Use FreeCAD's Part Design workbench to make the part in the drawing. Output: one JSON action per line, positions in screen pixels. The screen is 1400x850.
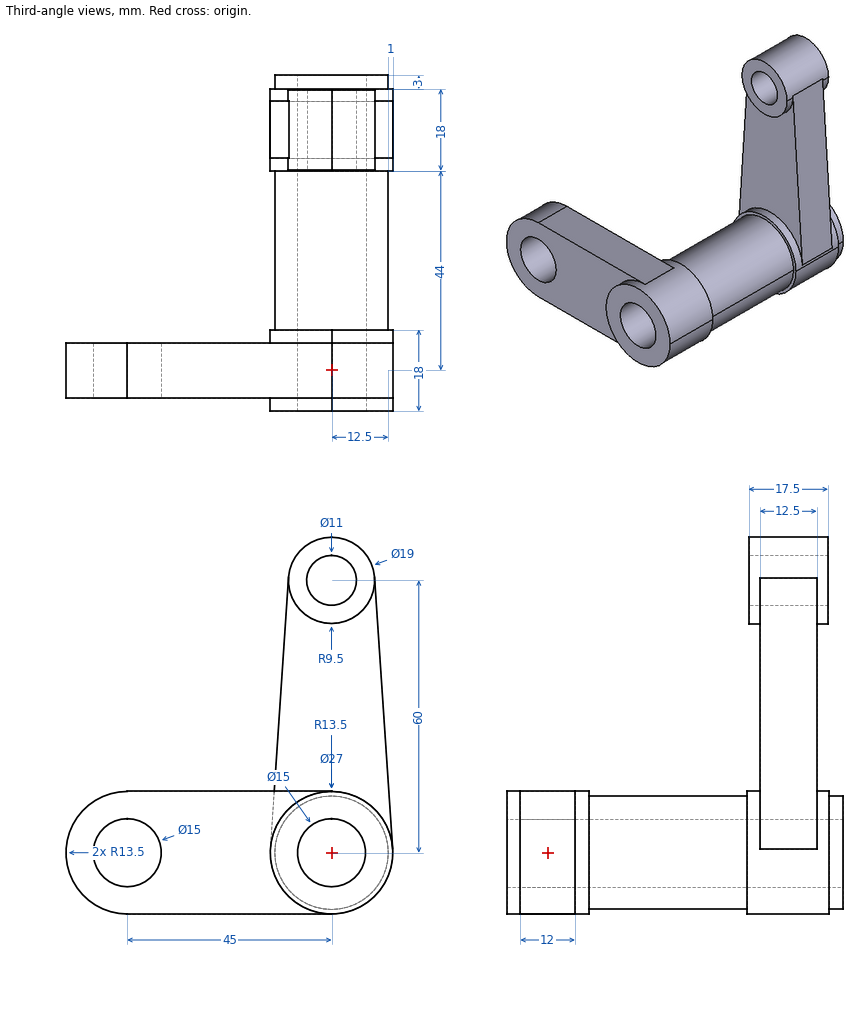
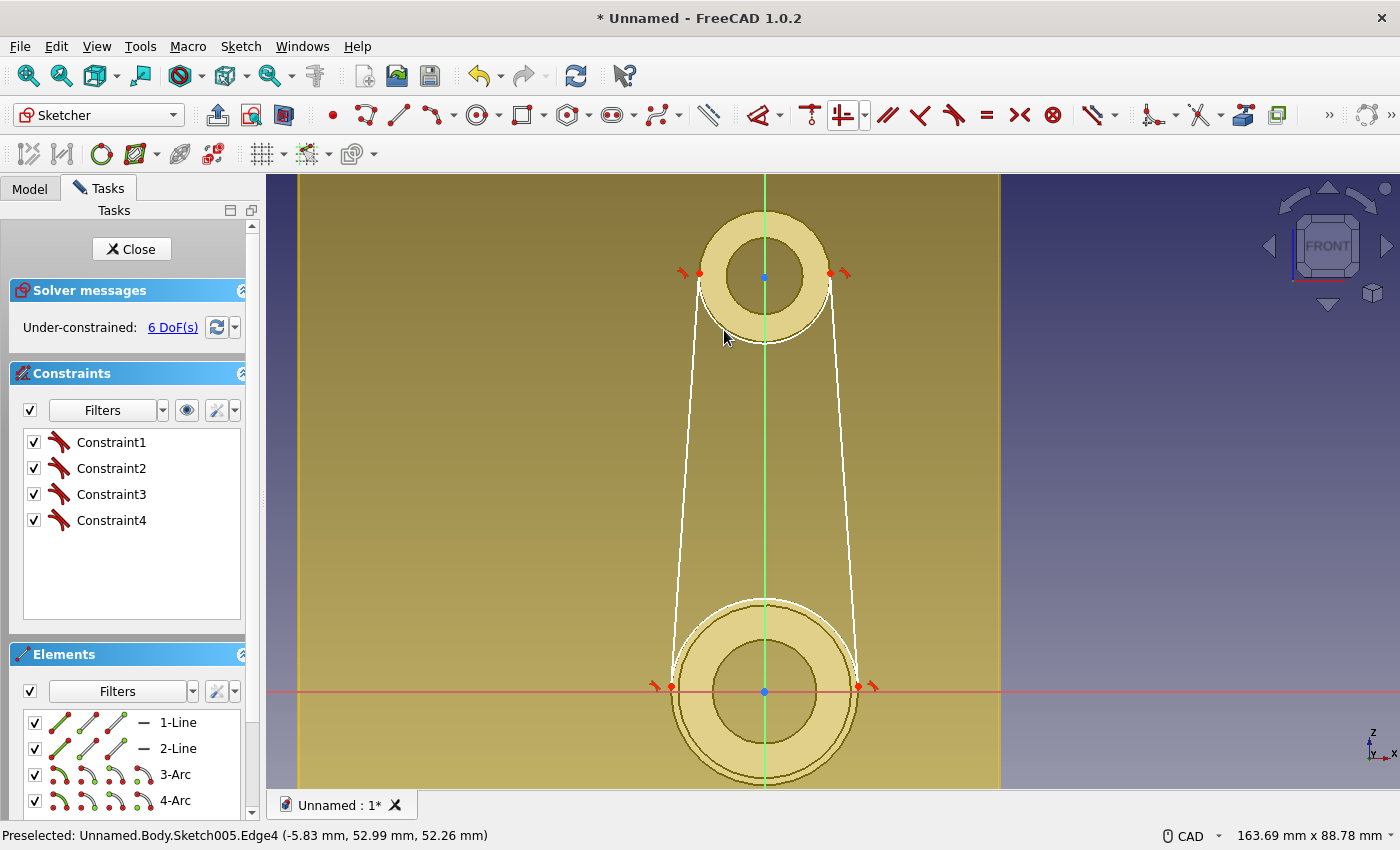
{"action": "left_click_drag", "start_coordinate": [755, 682], "coordinate": [775, 702]}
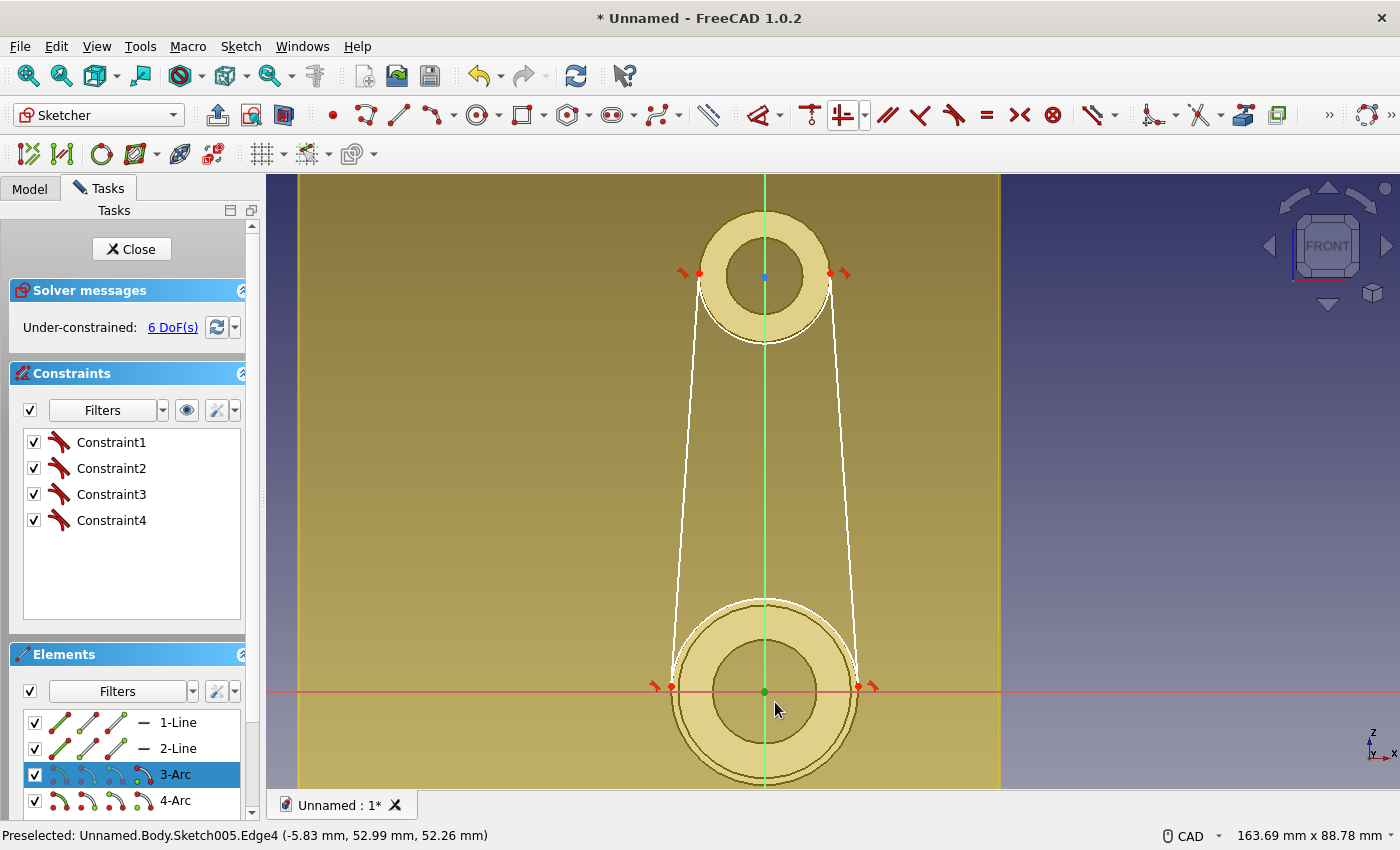
{"action": "left_click", "coordinate": [810, 116]}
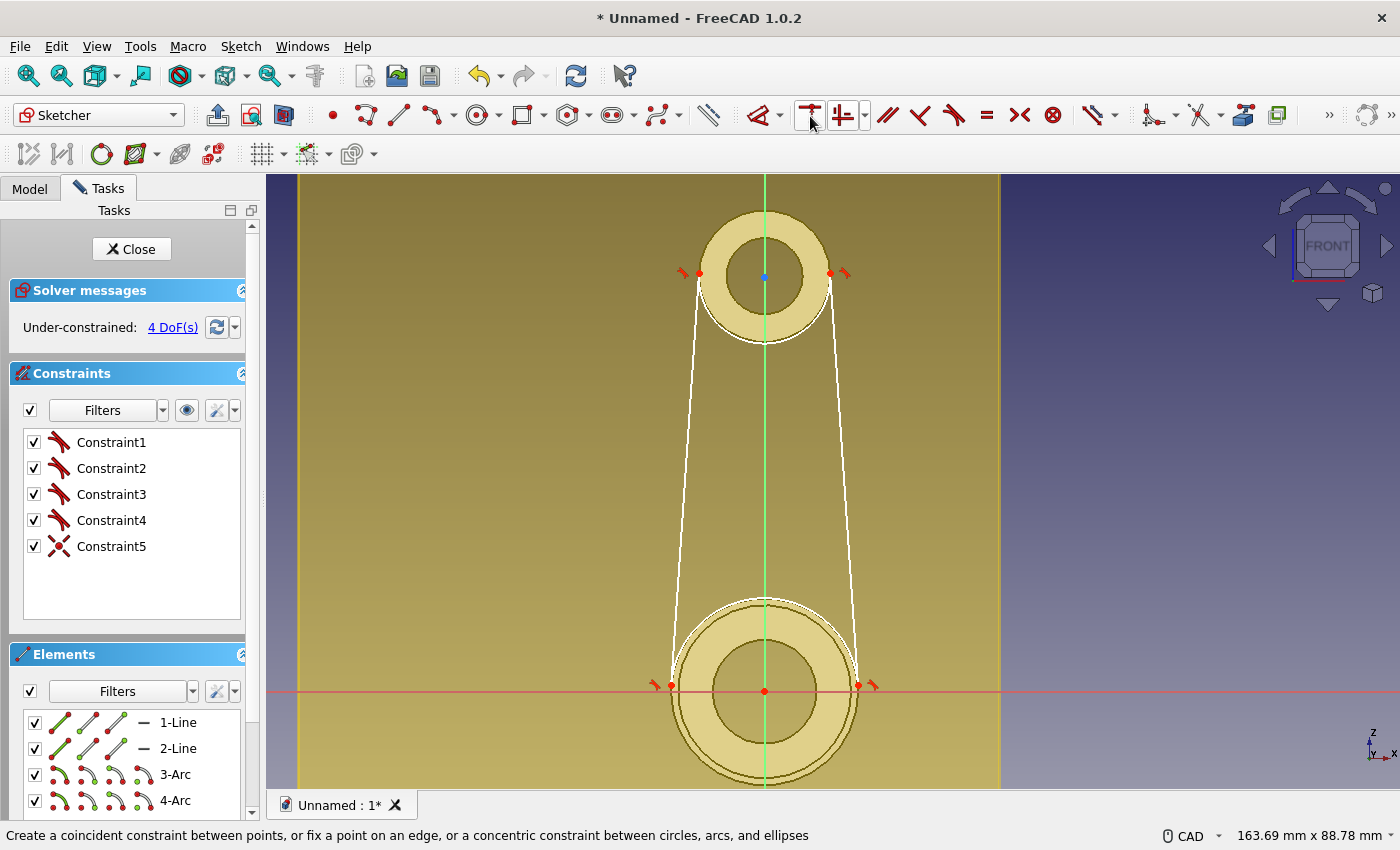
{"action": "left_click", "coordinate": [765, 278]}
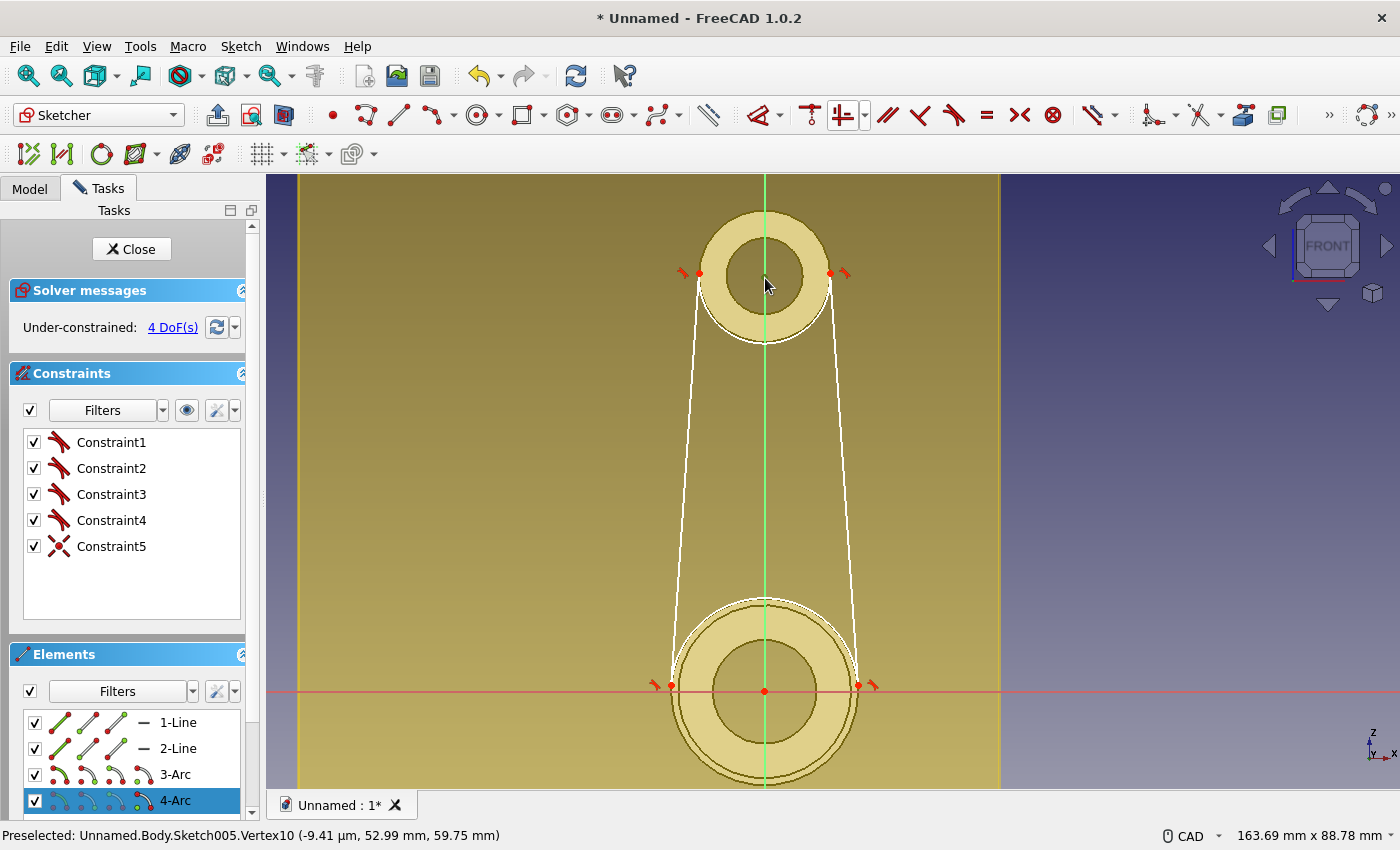
{"action": "left_click", "coordinate": [765, 641]}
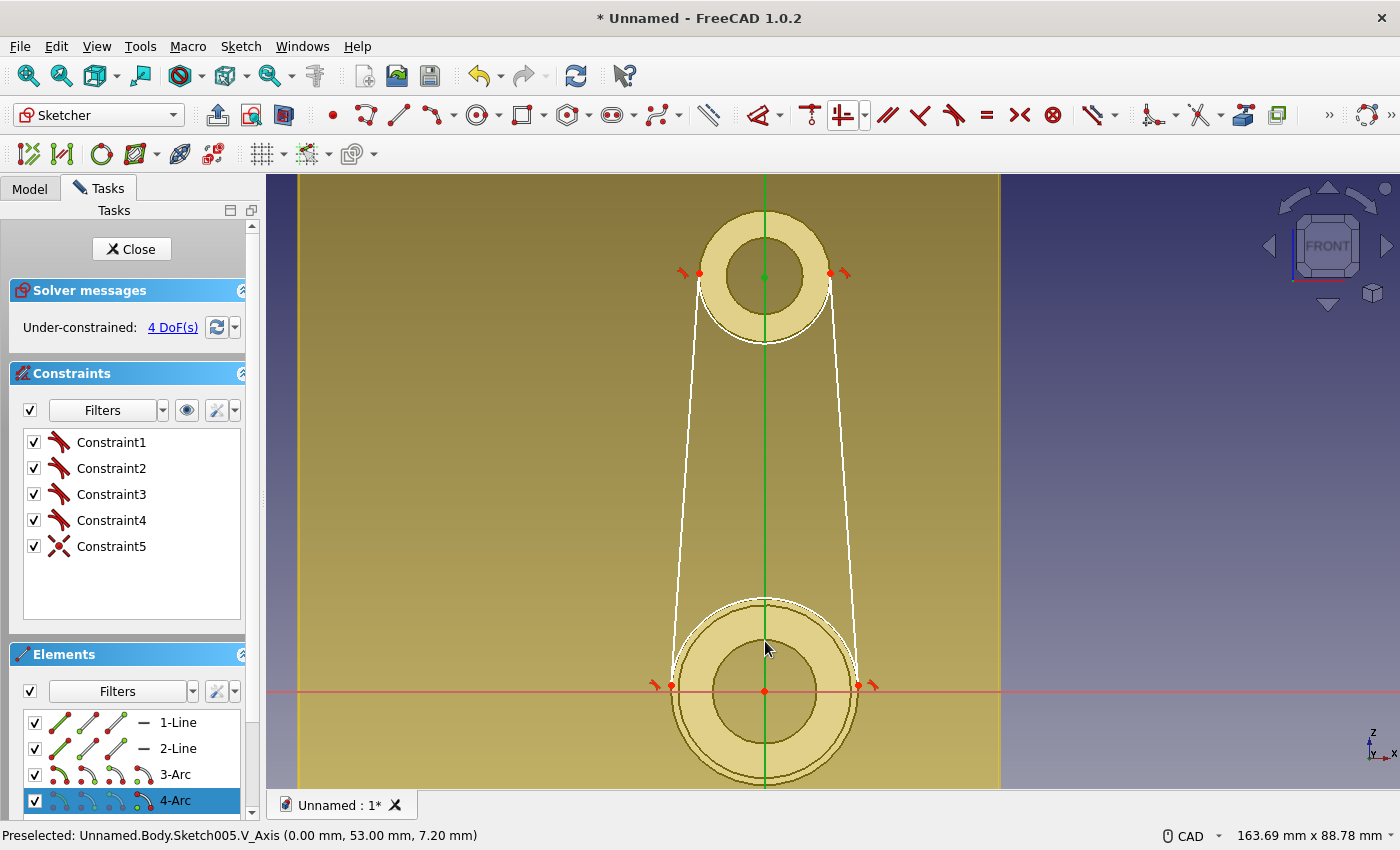
{"action": "key", "text": "c"}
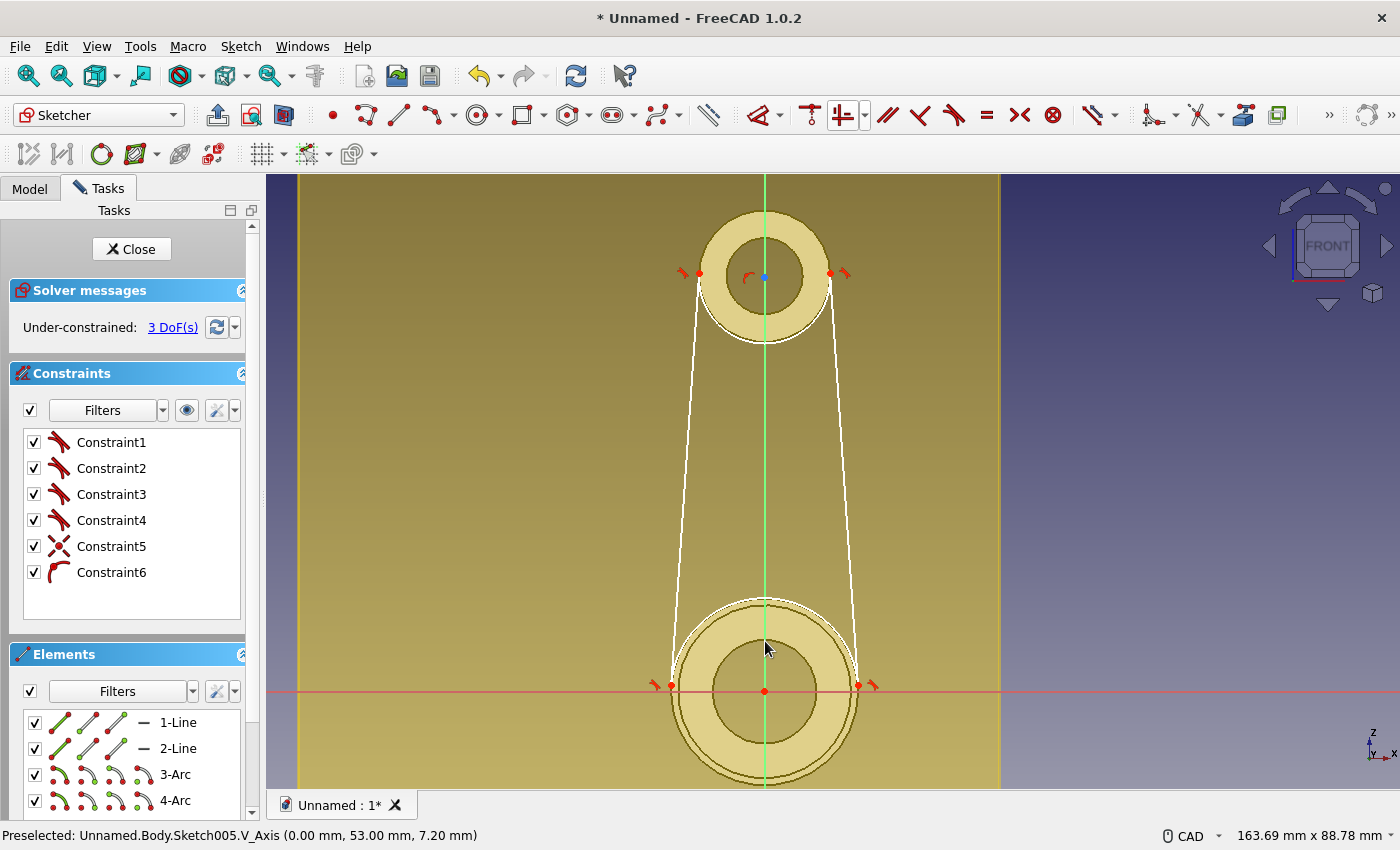
{"action": "key", "text": "d"}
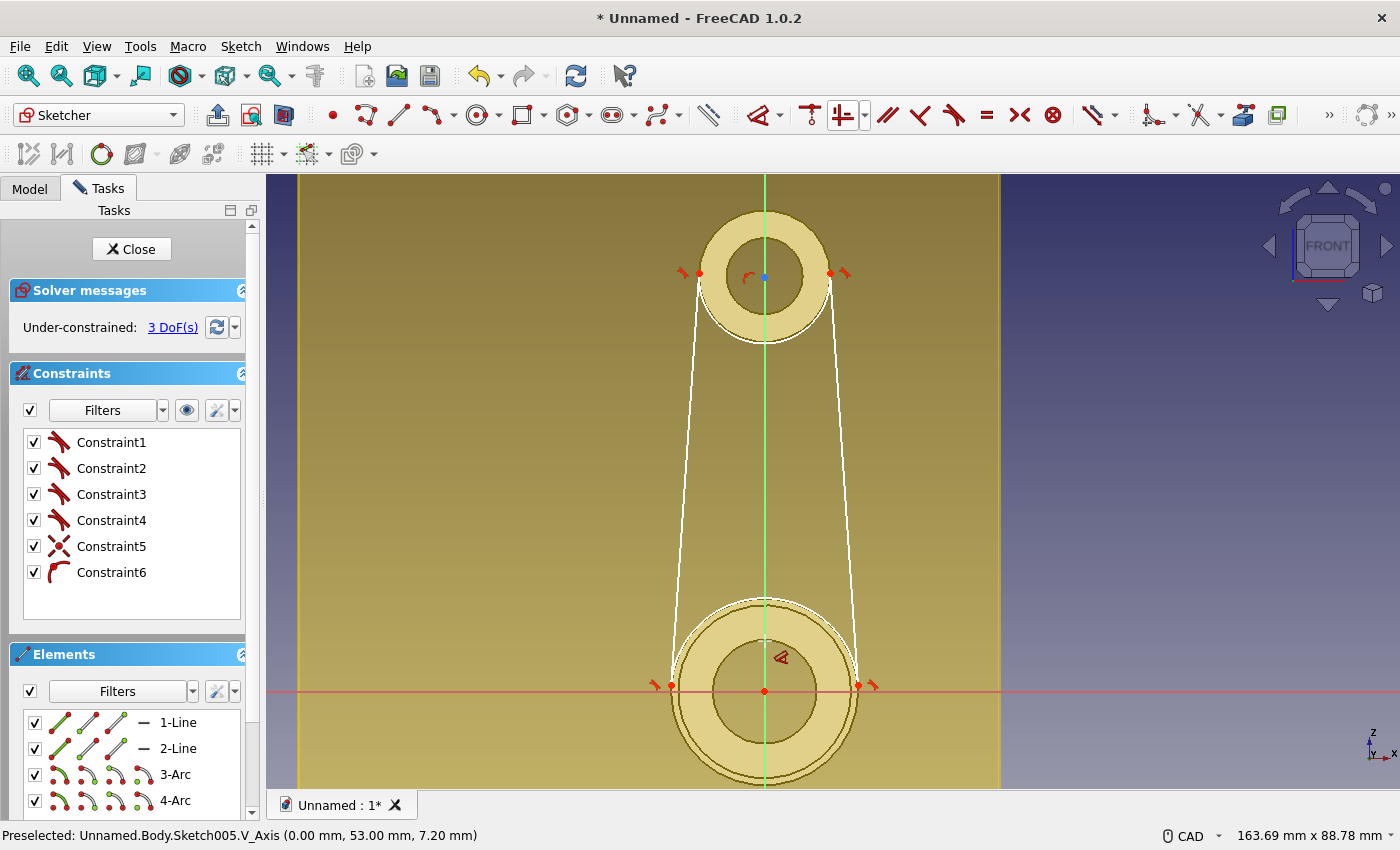
{"action": "left_click", "coordinate": [818, 615]}
{"action": "left_click", "coordinate": [836, 589]}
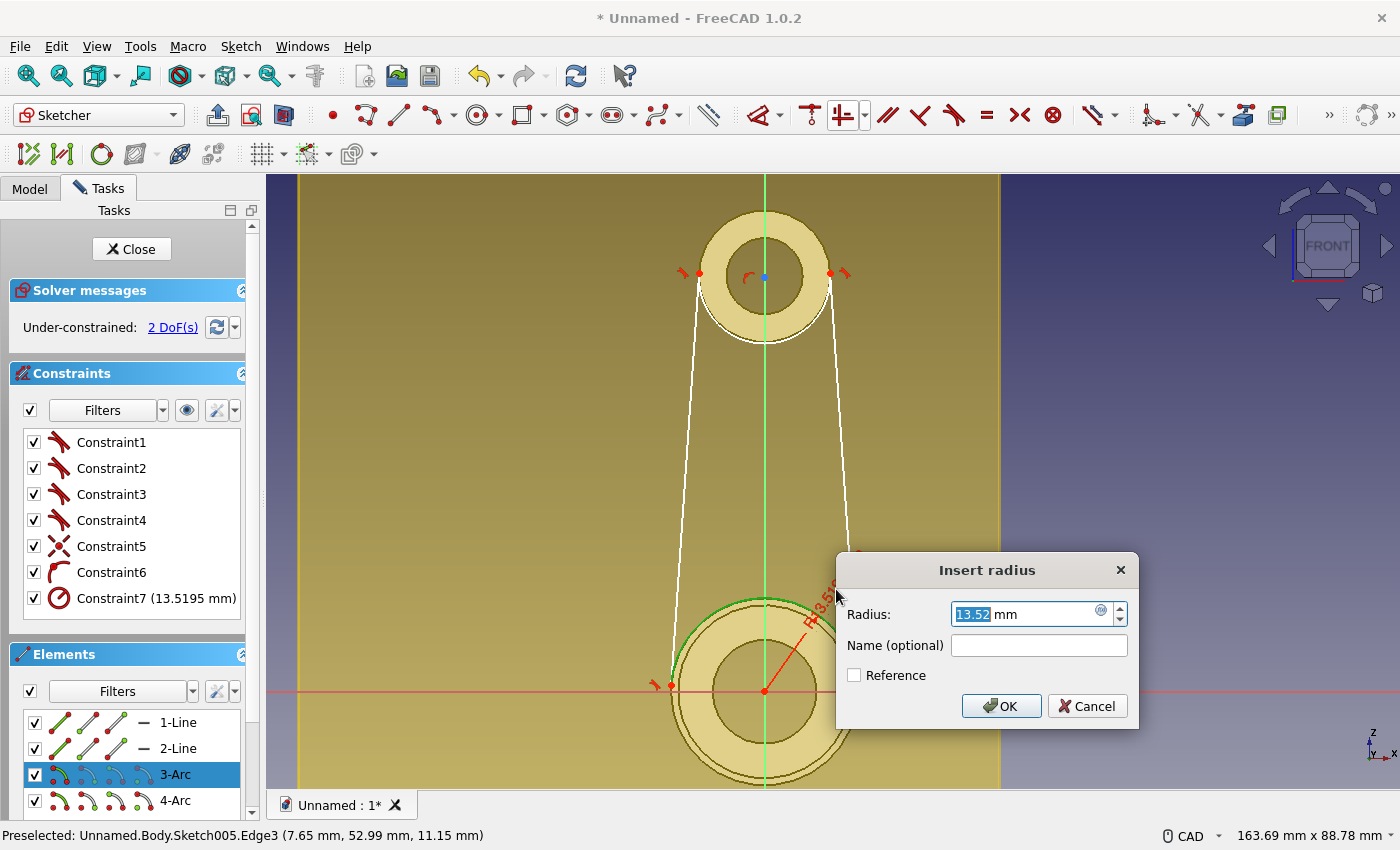
{"action": "type", "text": "13.5"}
{"action": "key", "text": "Return"}